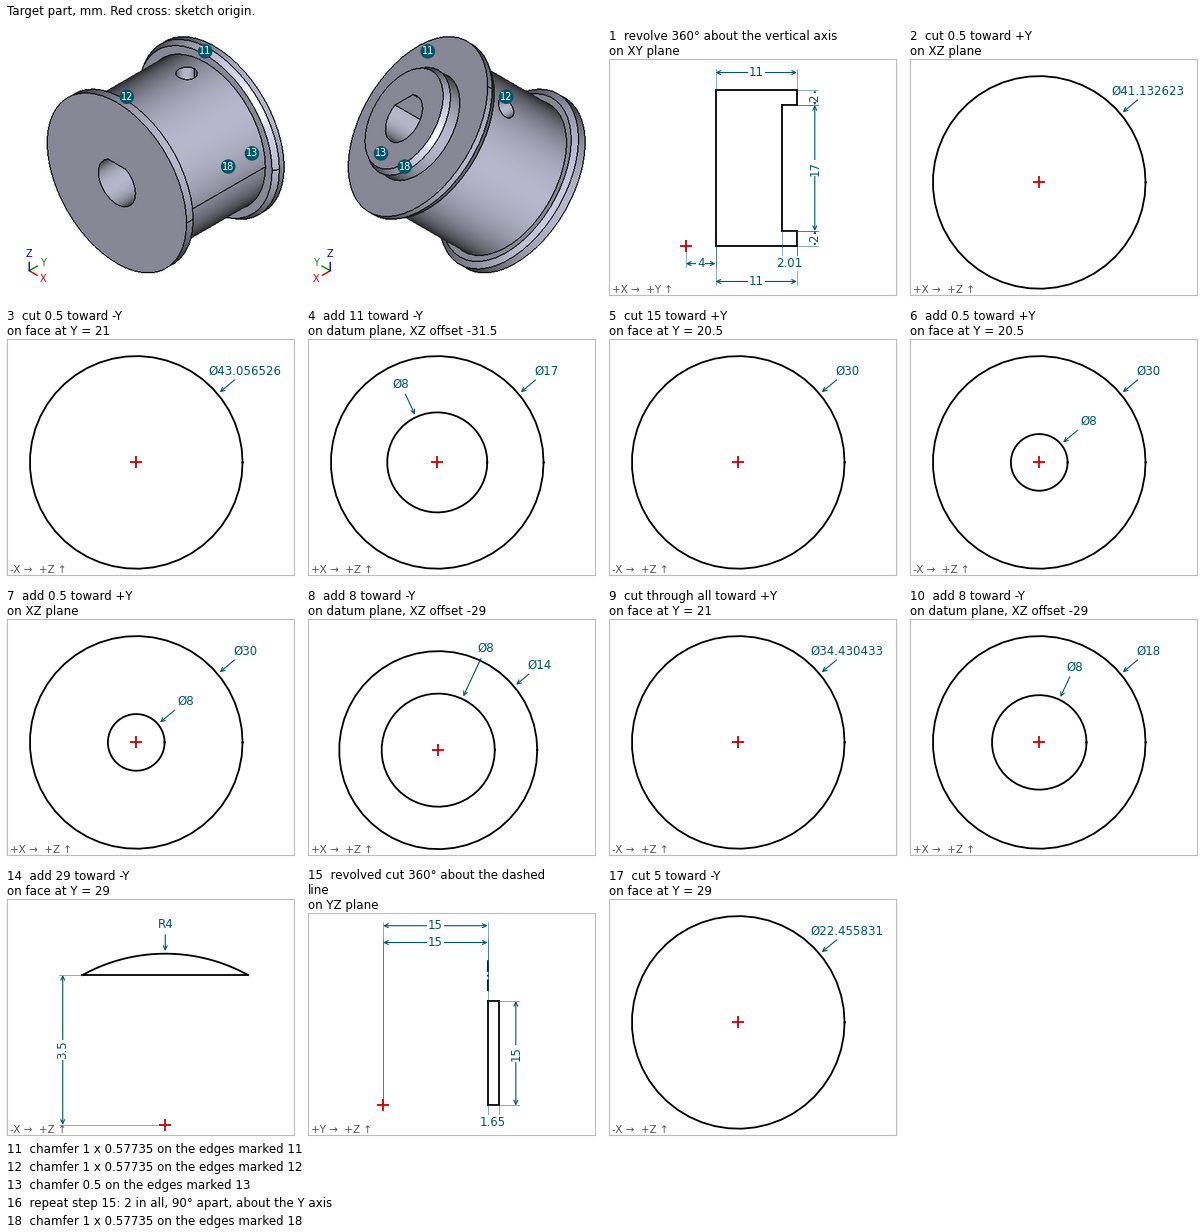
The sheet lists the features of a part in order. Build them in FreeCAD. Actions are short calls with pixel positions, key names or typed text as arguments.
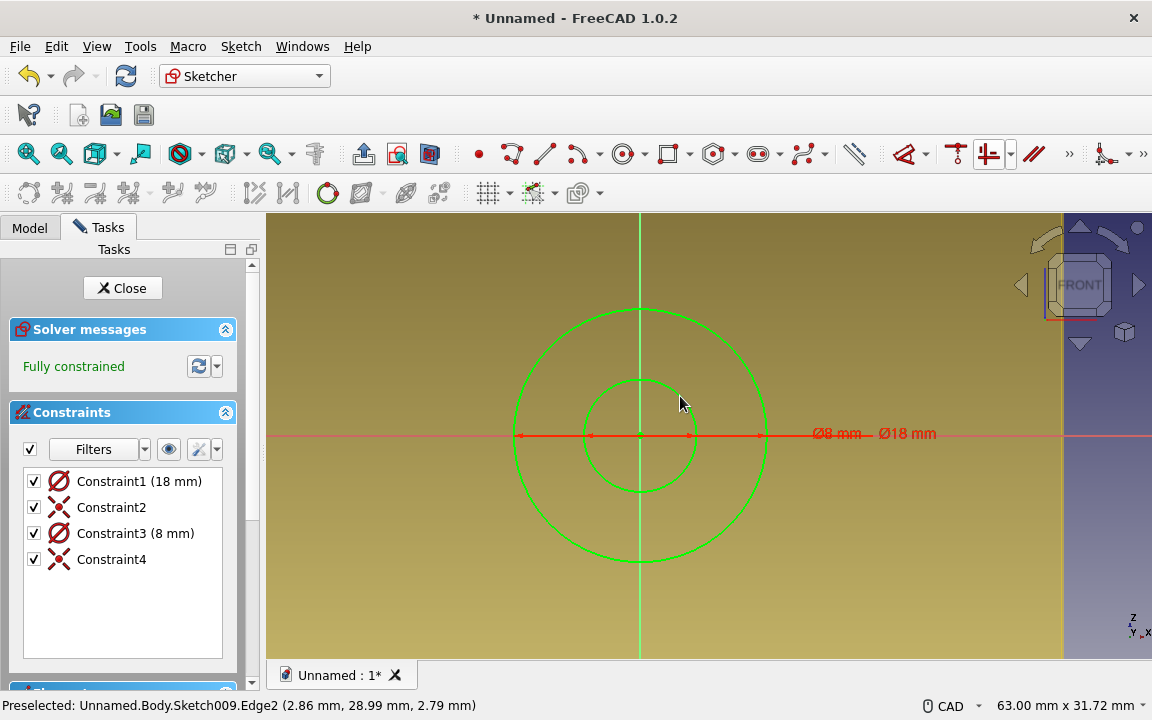
click(123, 288)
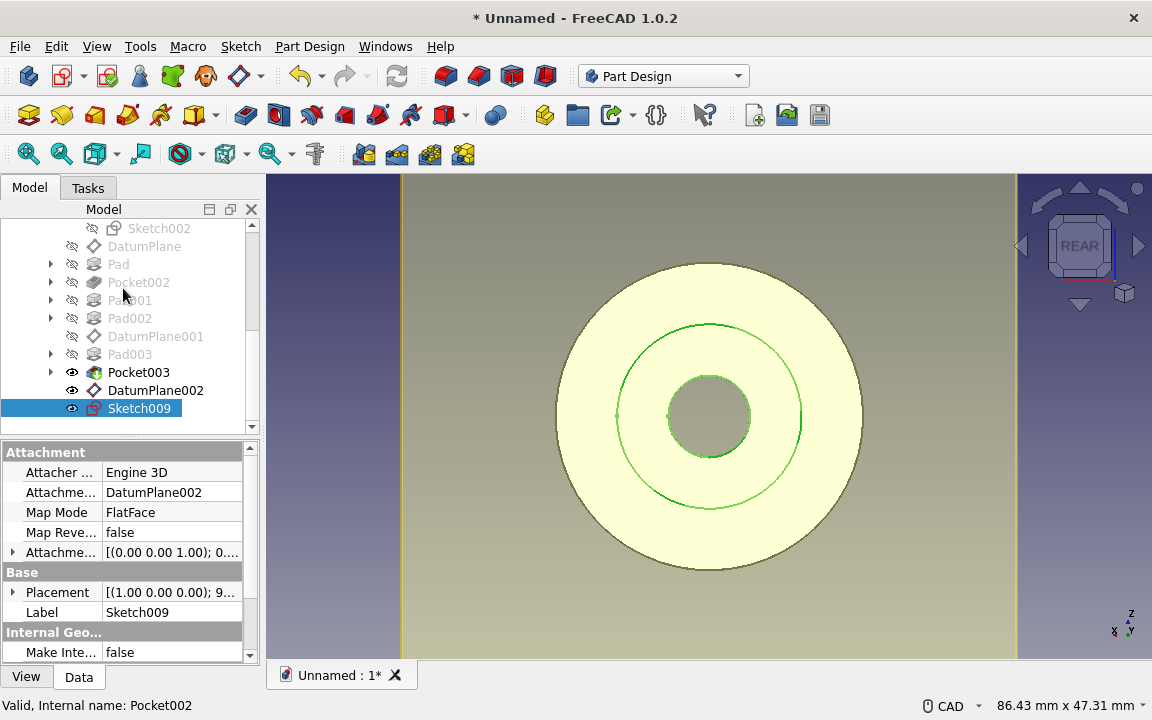
click(29, 116)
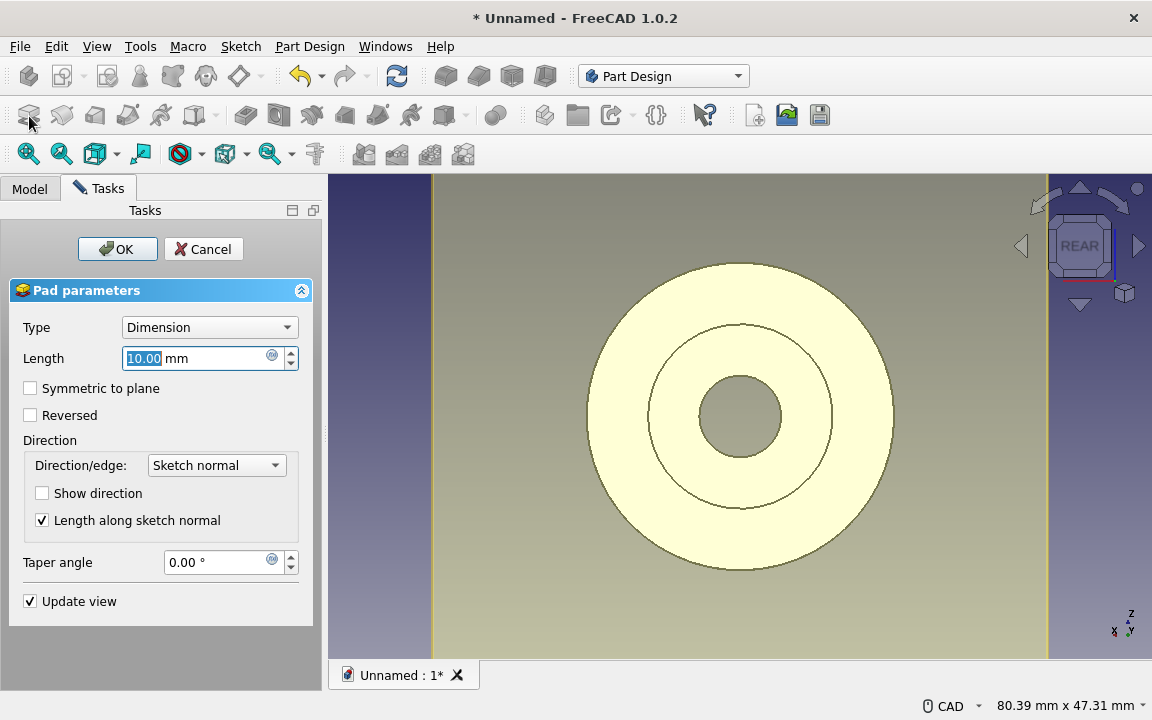
text(8)
key(Tab)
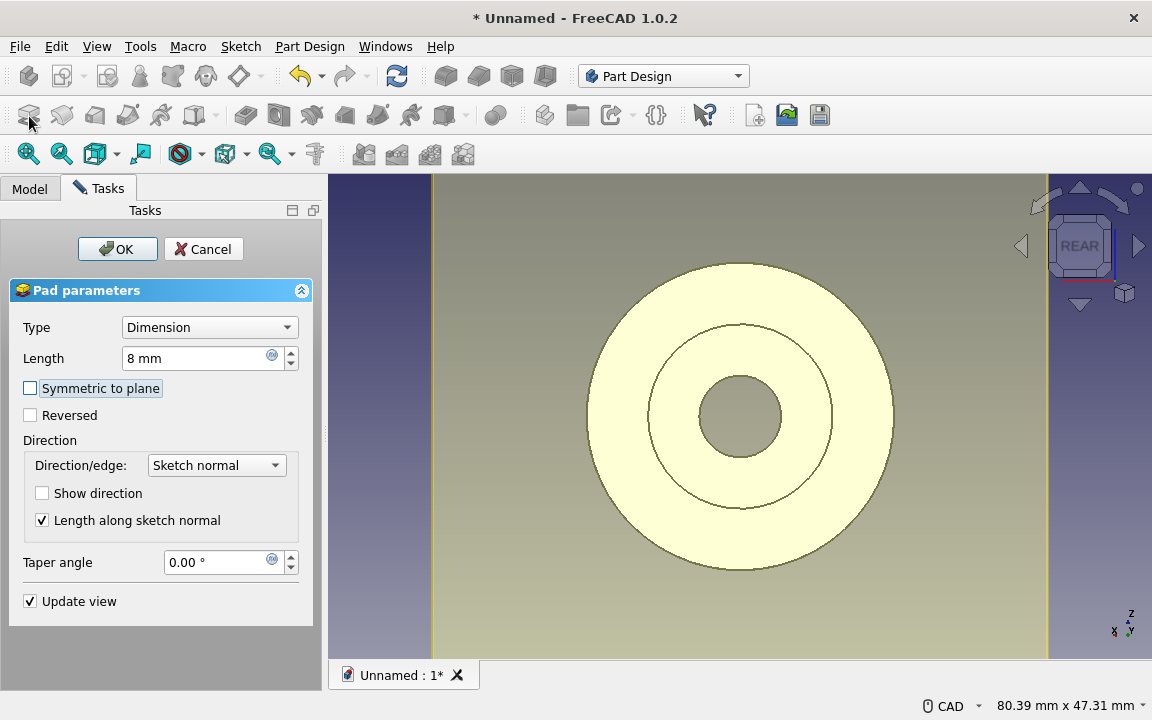
click(118, 249)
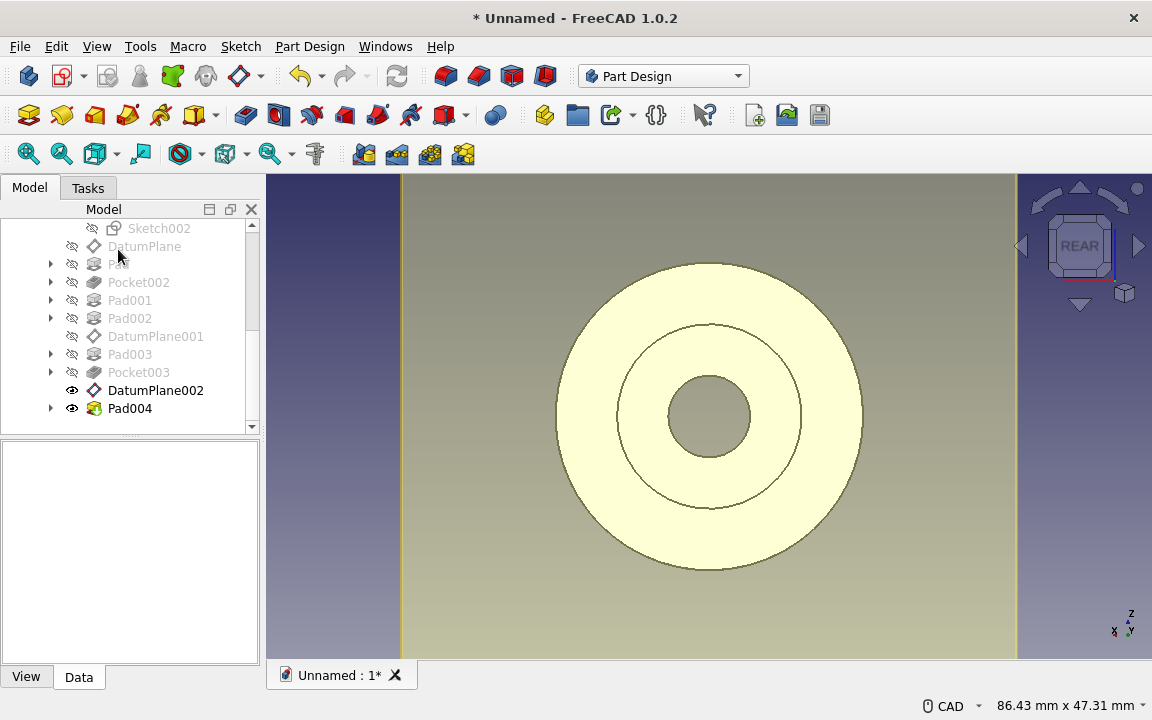
click(117, 390)
key(space)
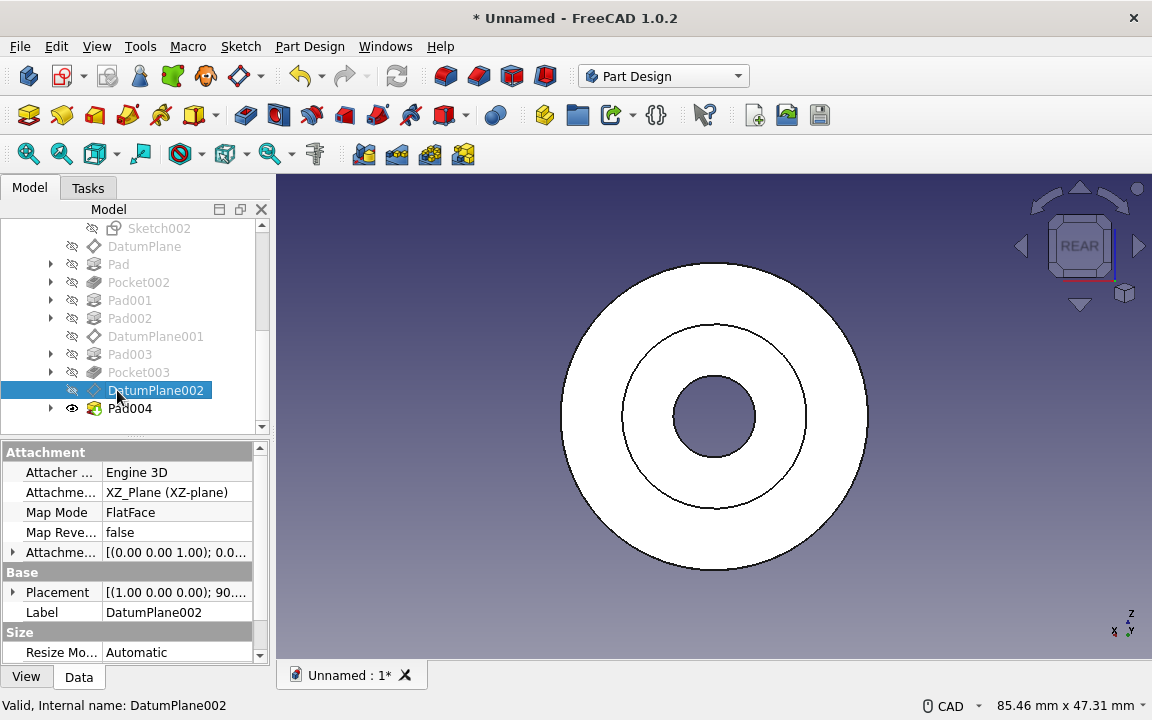
key(0)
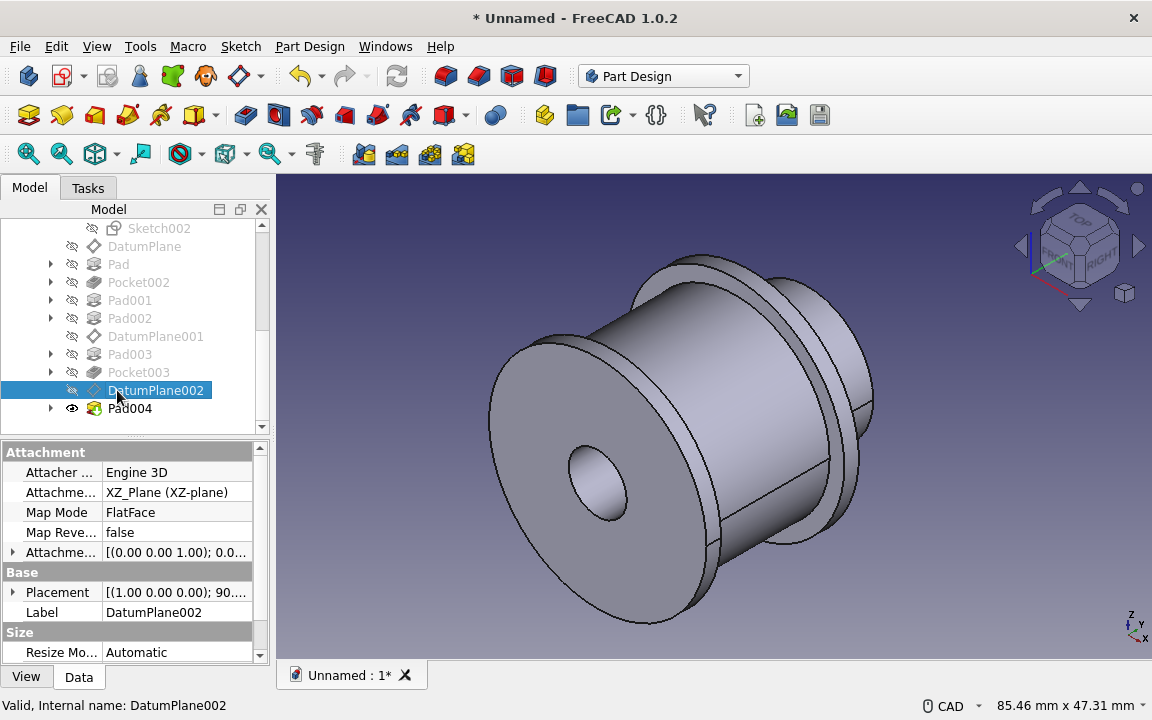
click(29, 154)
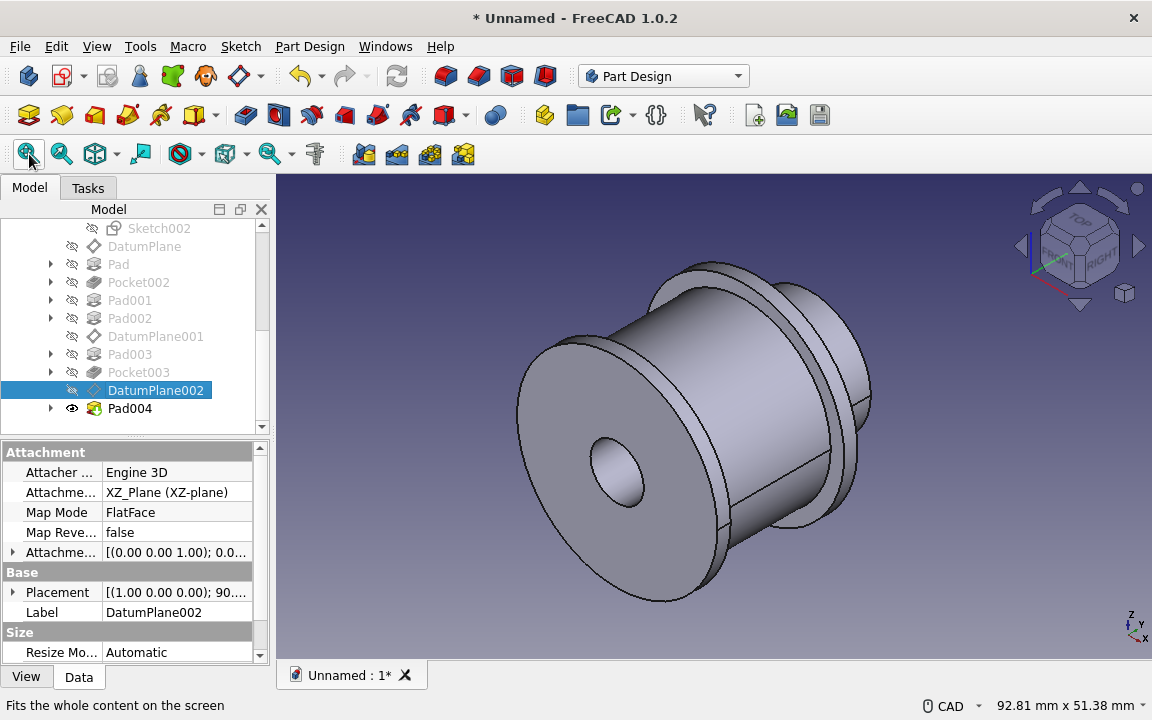
click(744, 283)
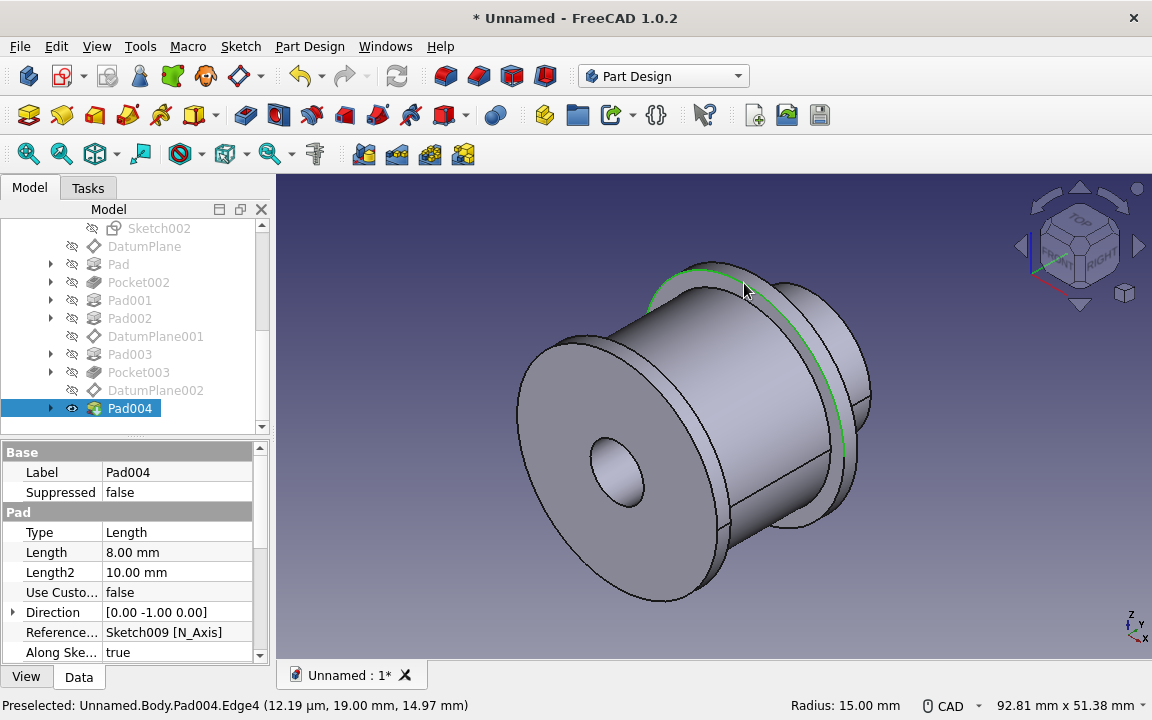
click(479, 76)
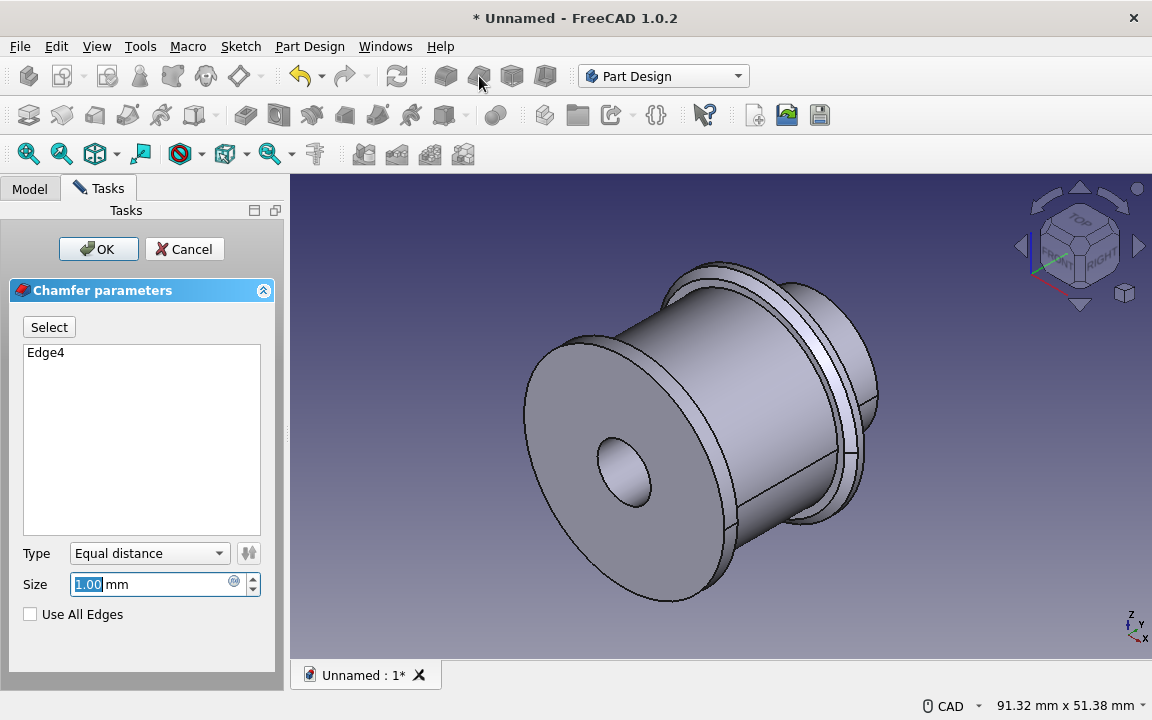
text(1)
key(Tab)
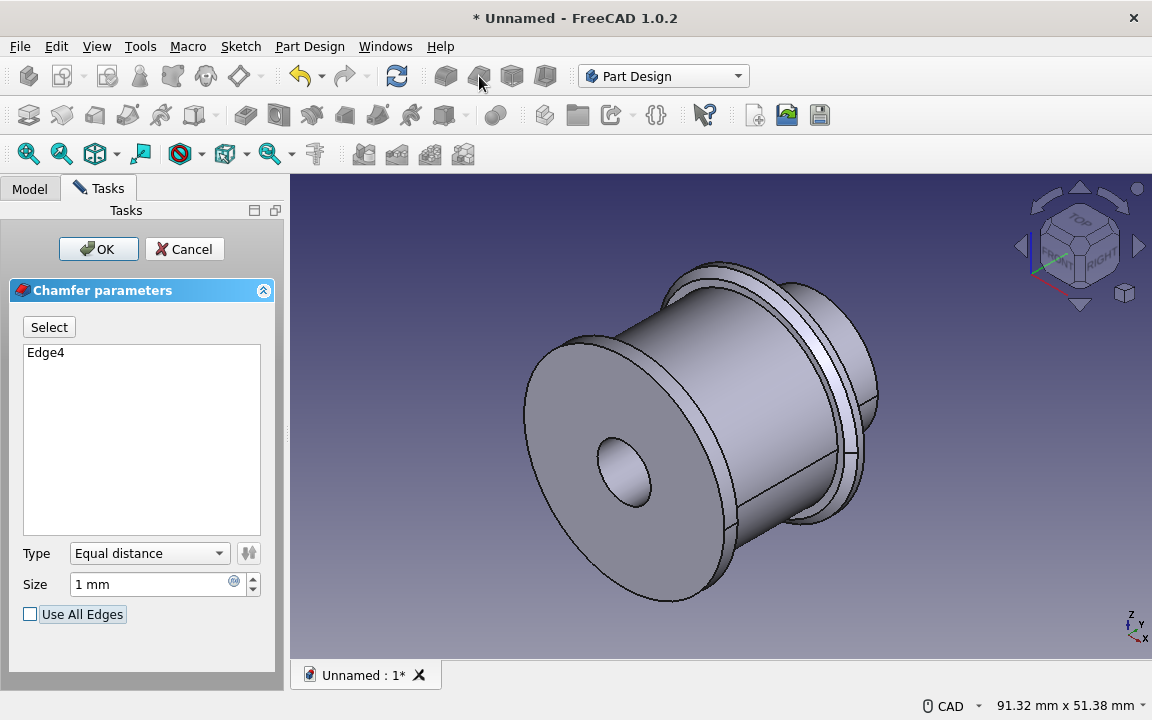
click(150, 554)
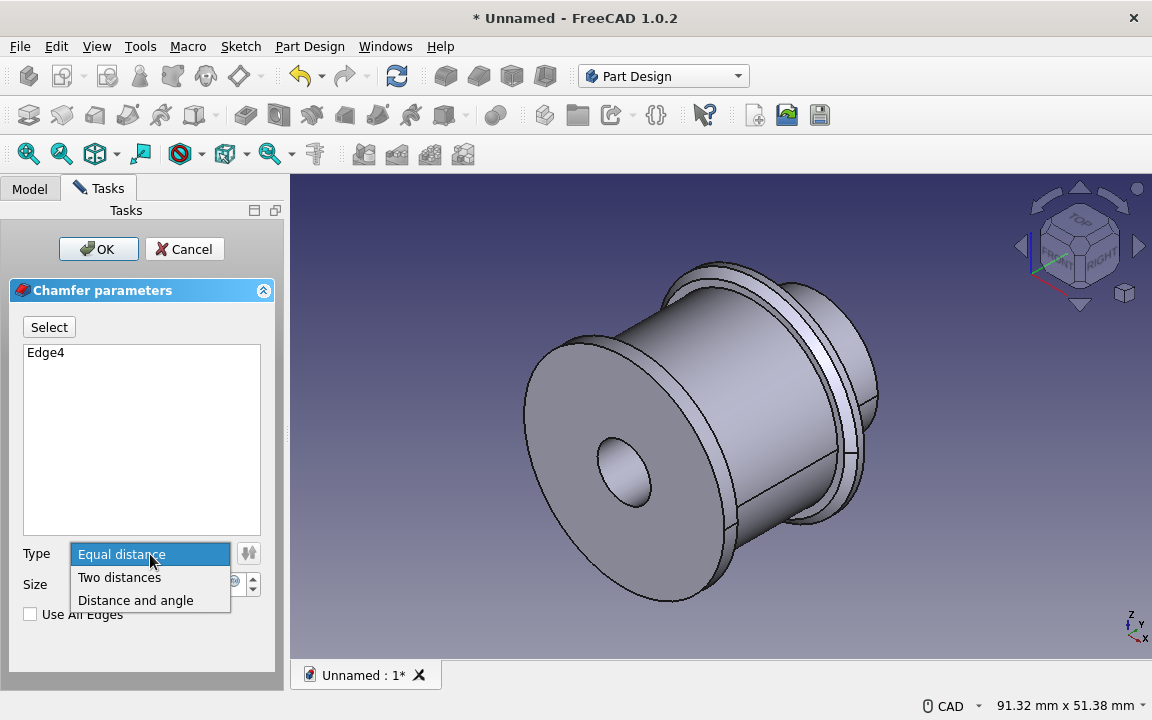
click(148, 578)